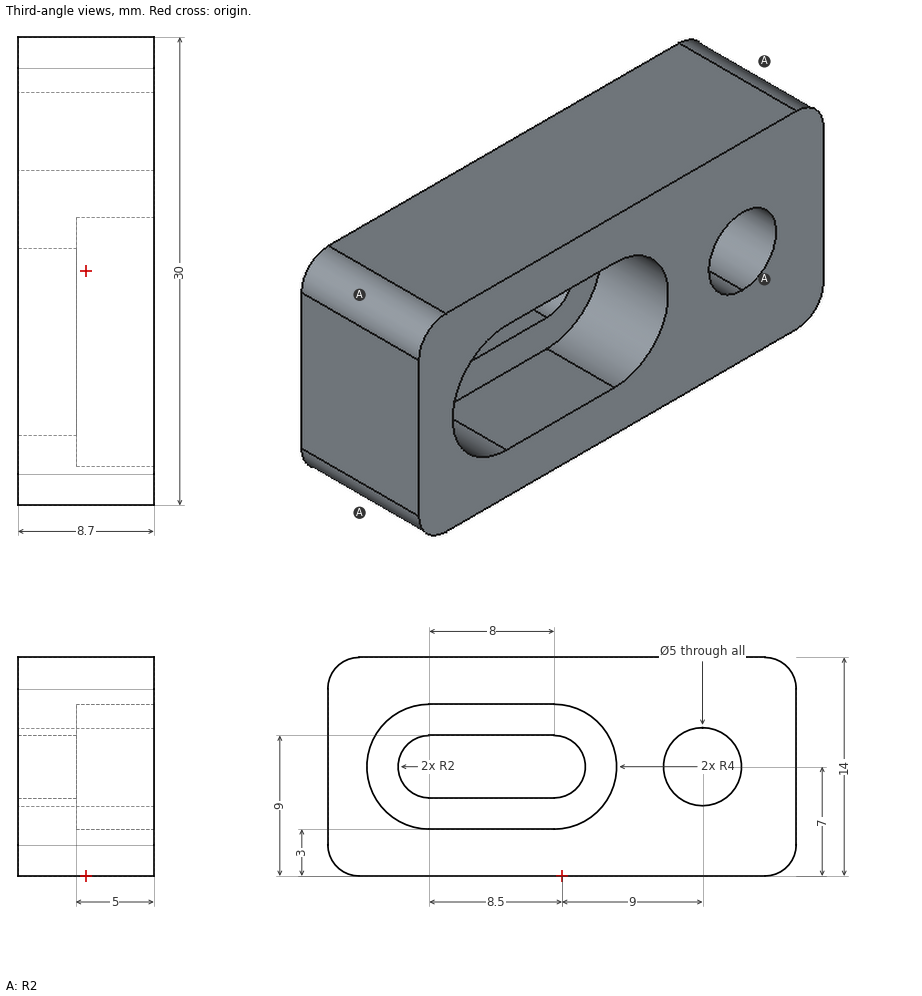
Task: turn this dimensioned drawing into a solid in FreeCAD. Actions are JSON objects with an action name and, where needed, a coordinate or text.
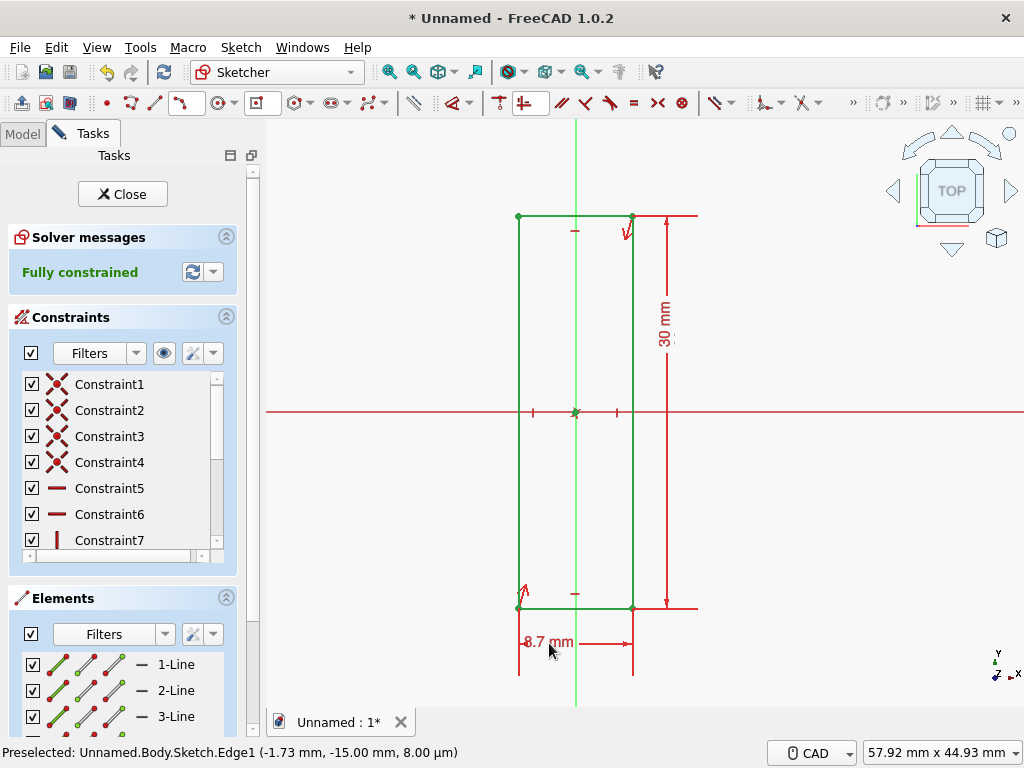
{"action": "left_click", "coordinate": [123, 194]}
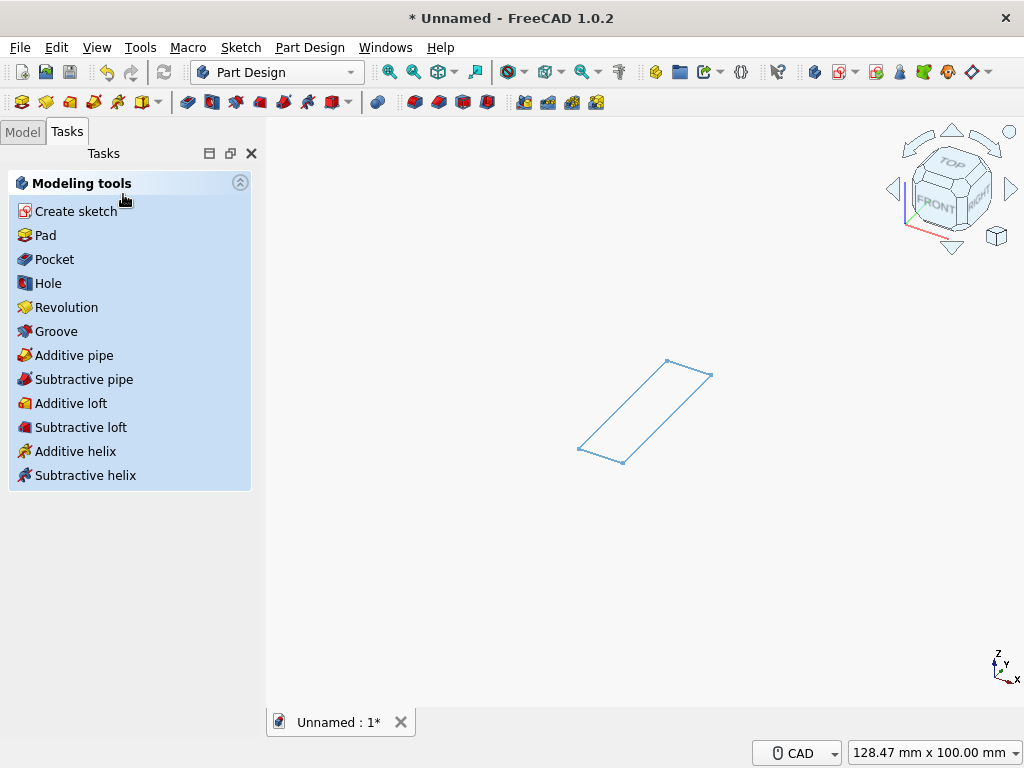
{"action": "left_click", "coordinate": [22, 102]}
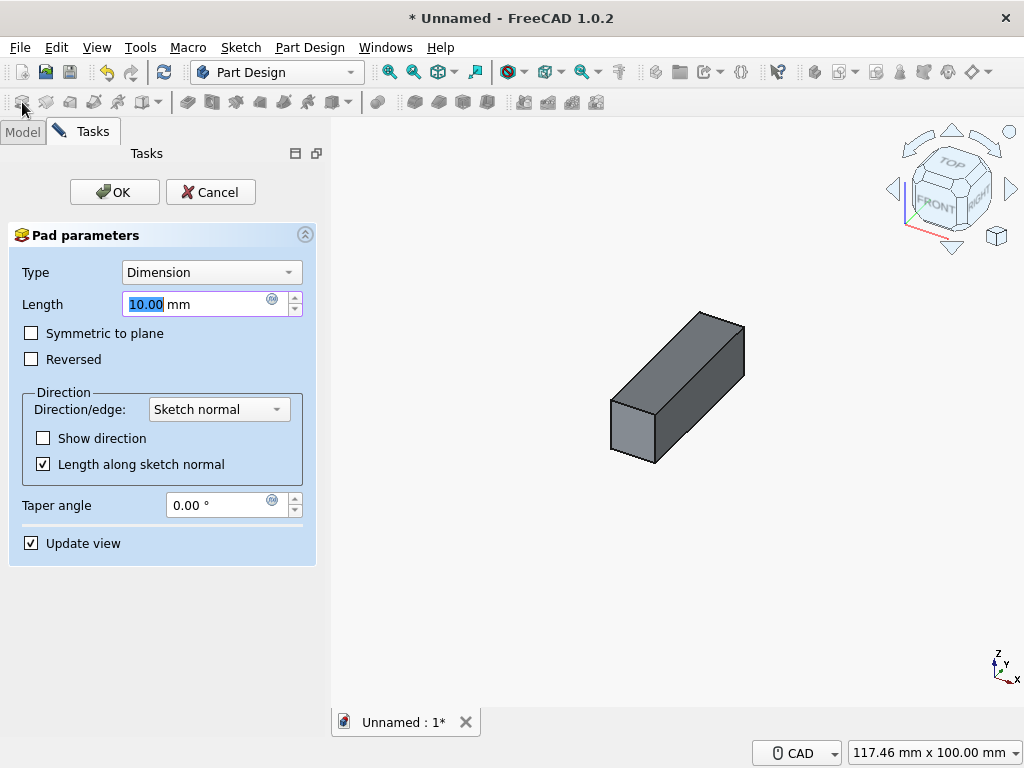
{"action": "type", "text": "14"}
{"action": "key", "text": "Tab"}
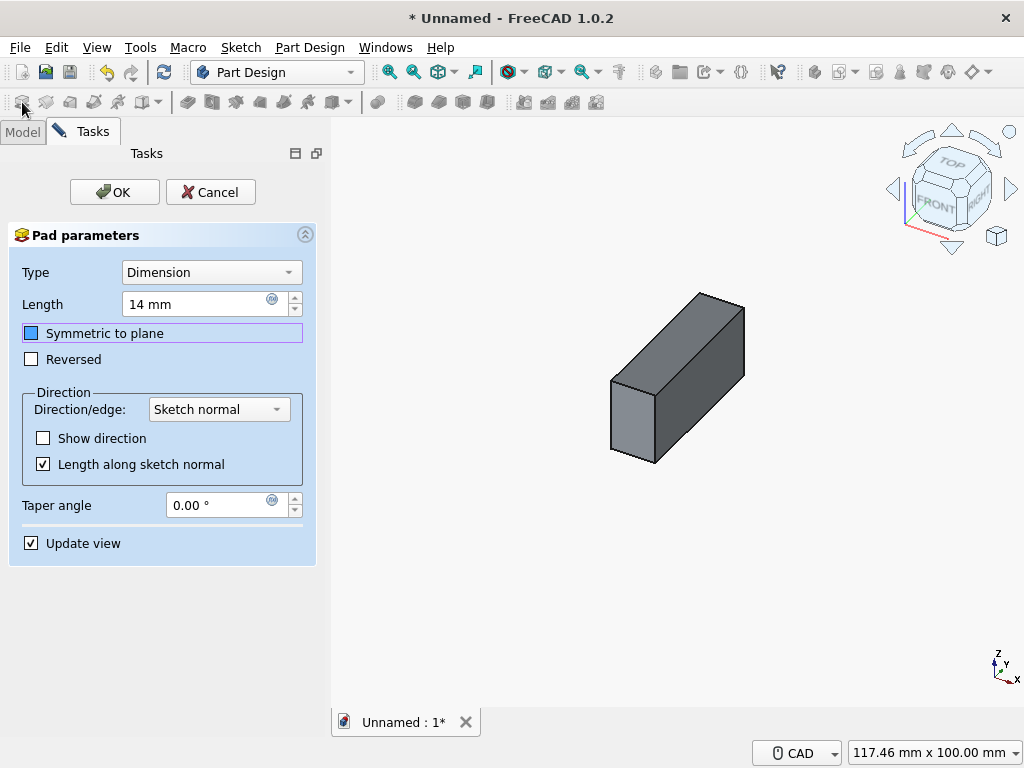
{"action": "left_click", "coordinate": [115, 192]}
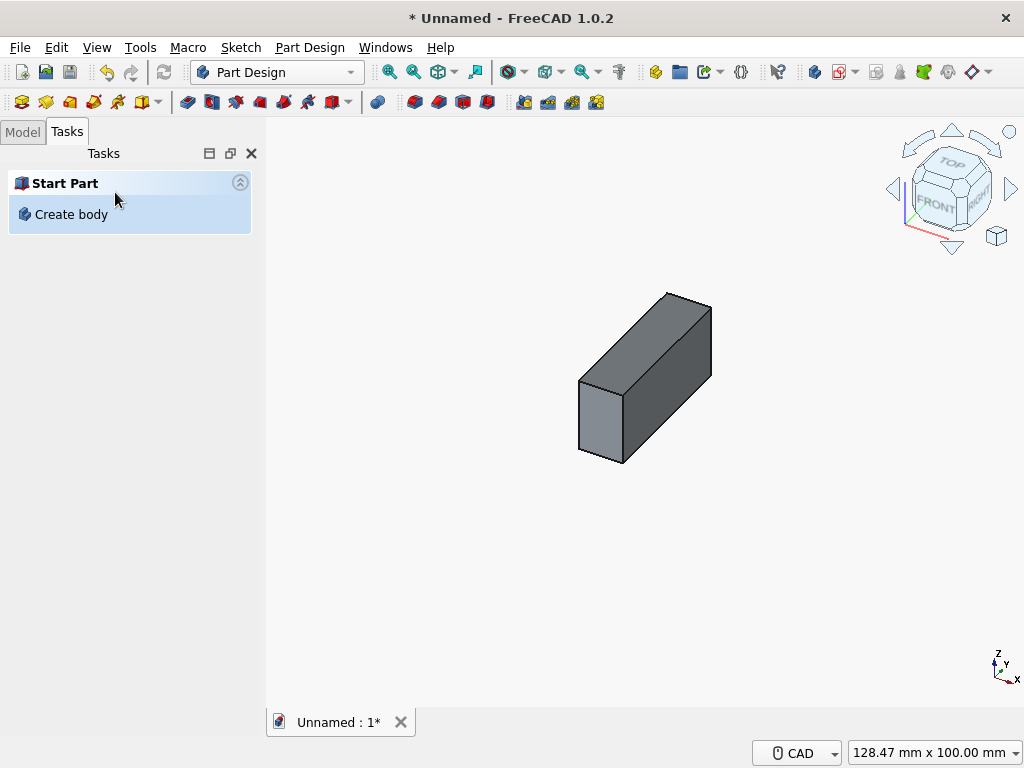
{"action": "left_click", "coordinate": [390, 72]}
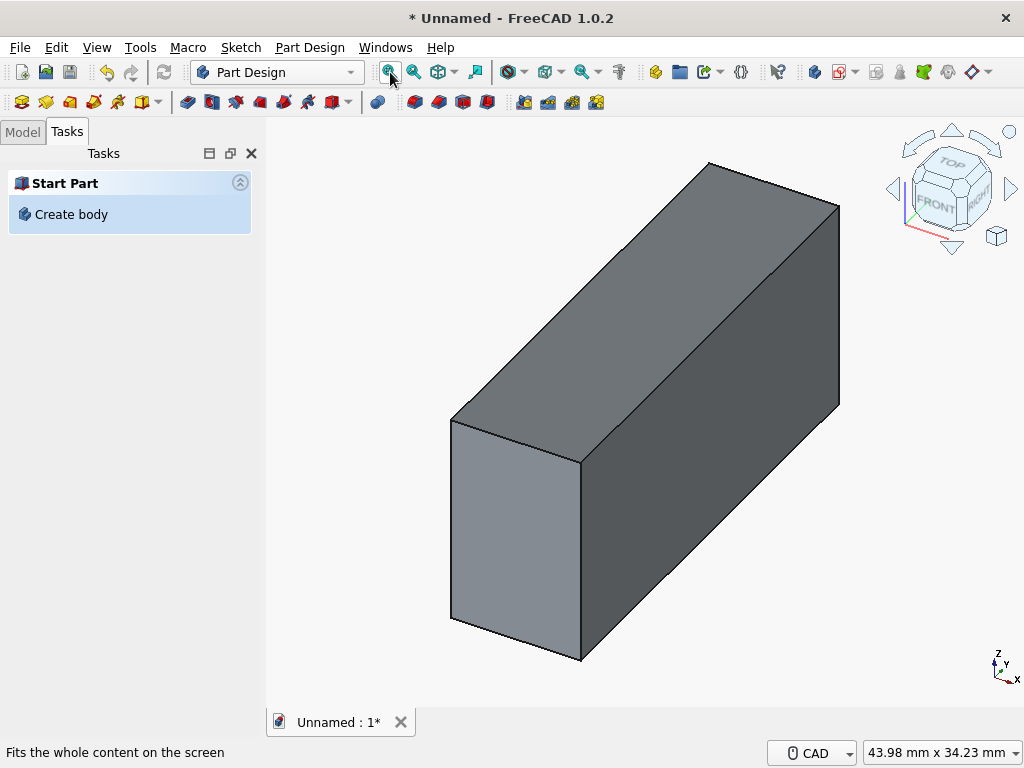
{"action": "left_click", "coordinate": [747, 396]}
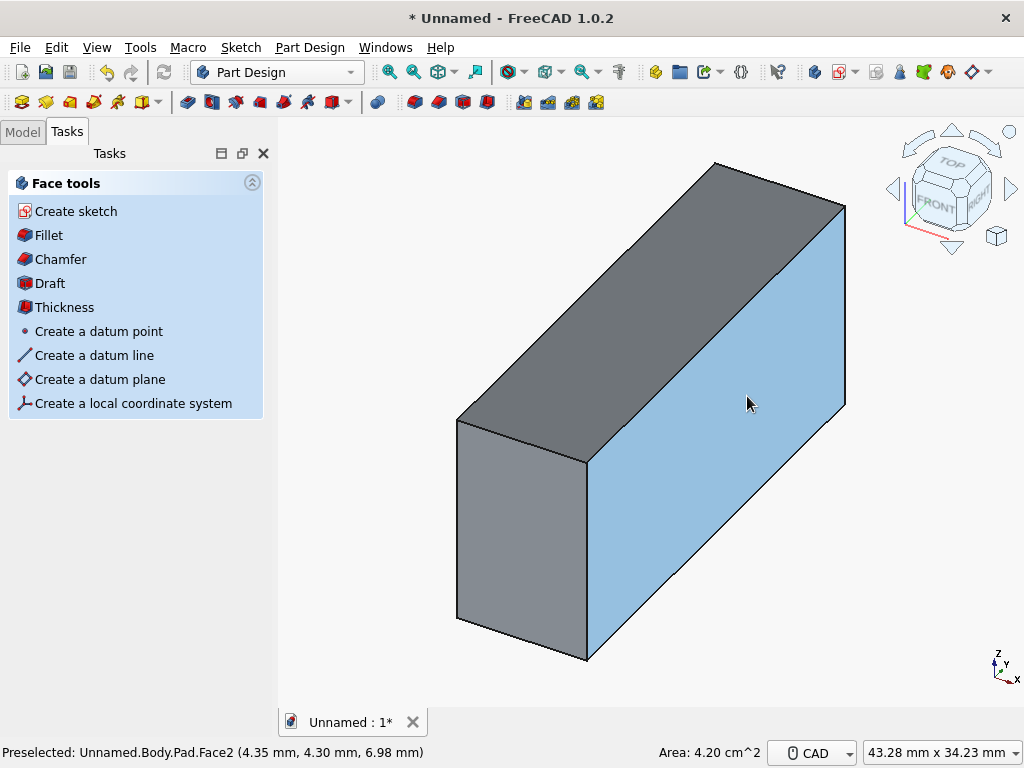
{"action": "left_click", "coordinate": [840, 72]}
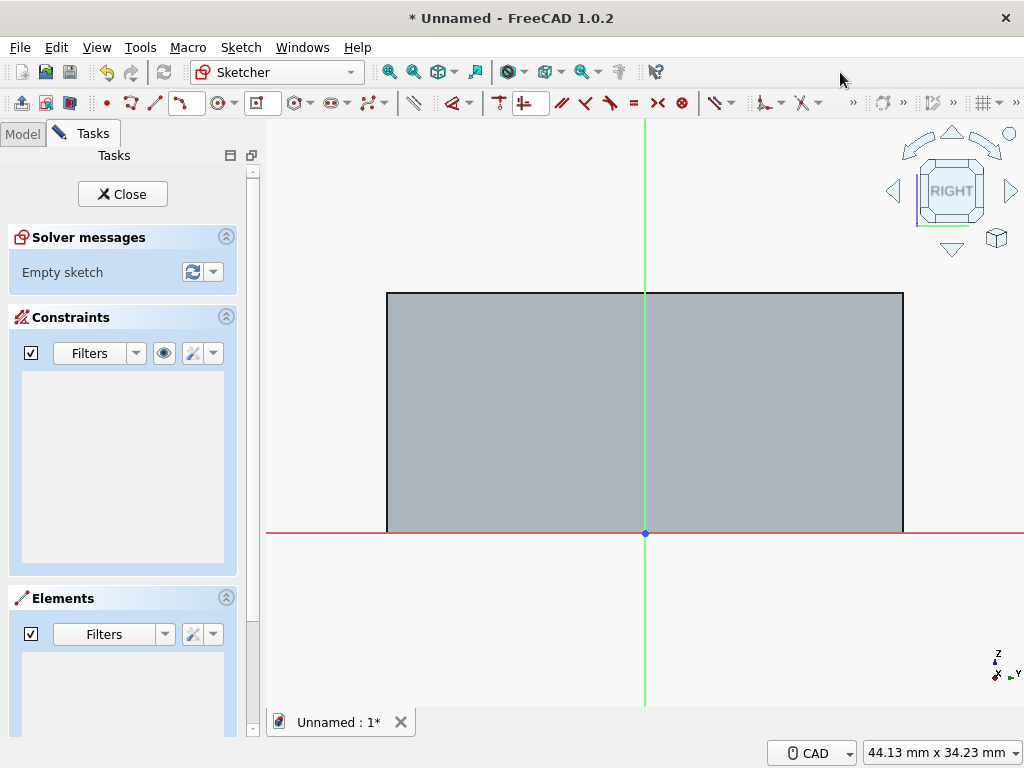
{"action": "scroll", "coordinate": [859, 483], "scroll_direction": "up", "scroll_amount": 4}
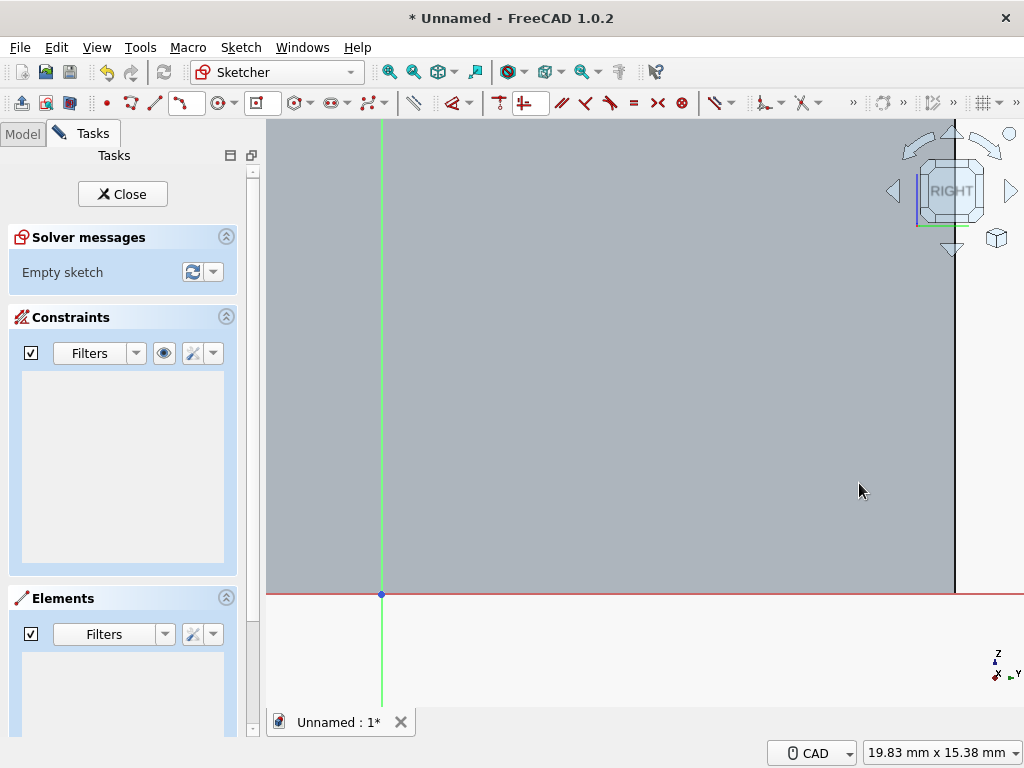
{"action": "left_click", "coordinate": [218, 104]}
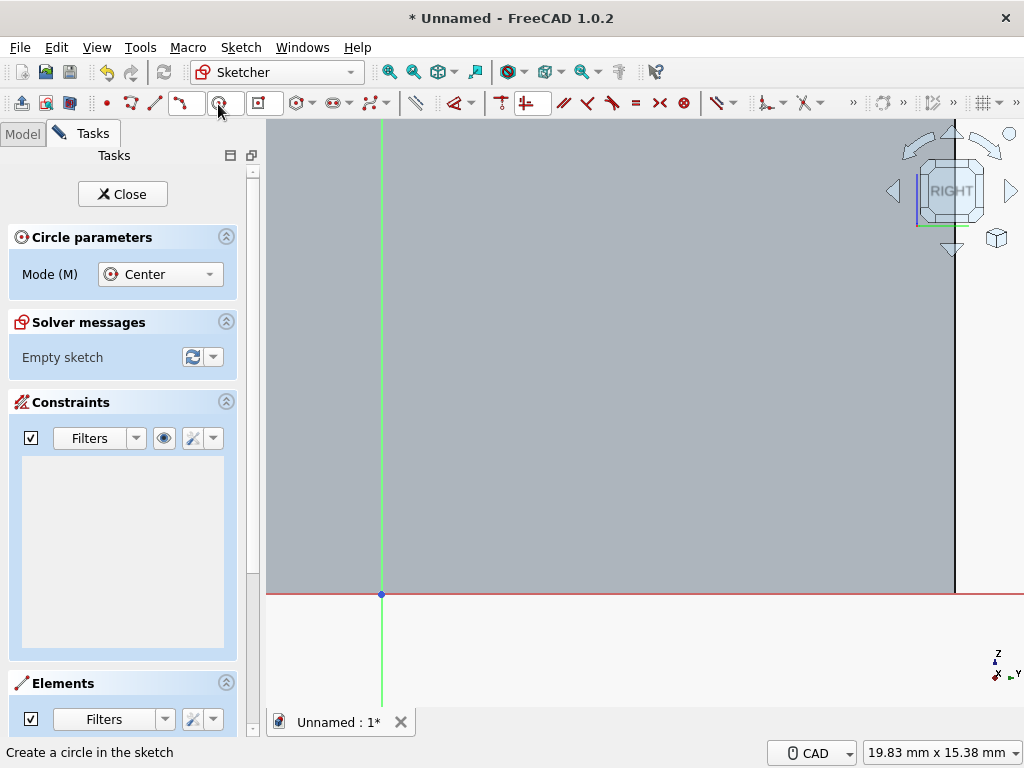
{"action": "left_click", "coordinate": [726, 326]}
{"action": "left_click", "coordinate": [793, 259]}
{"action": "key", "text": "Escape"}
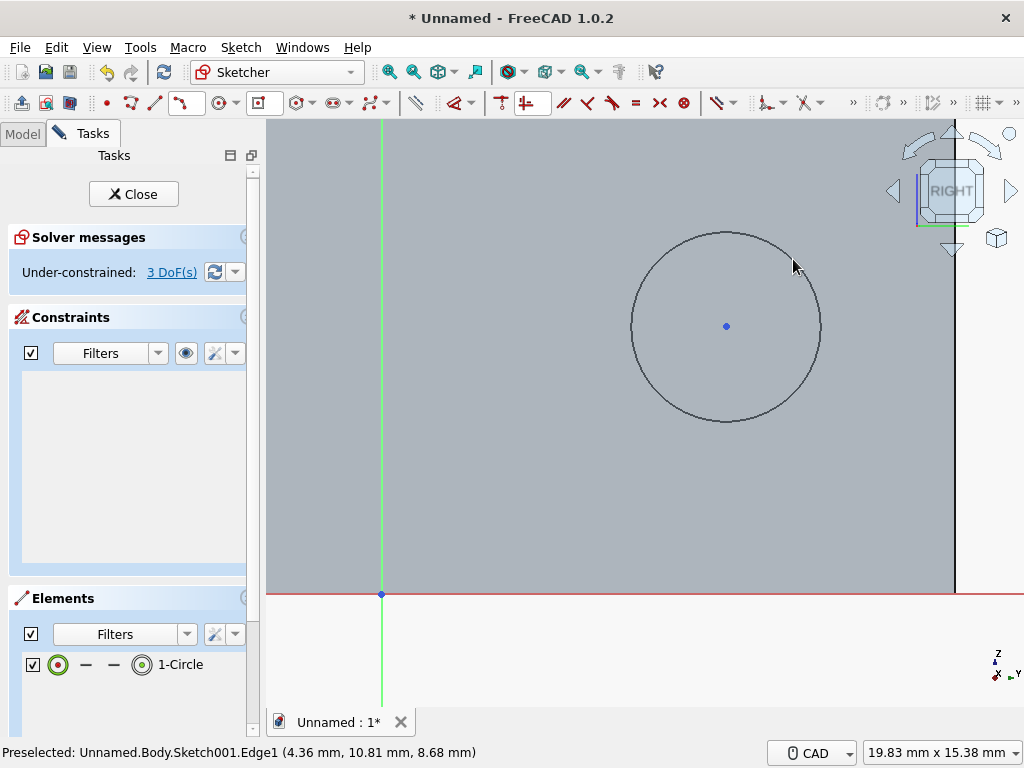
{"action": "left_click", "coordinate": [454, 104]}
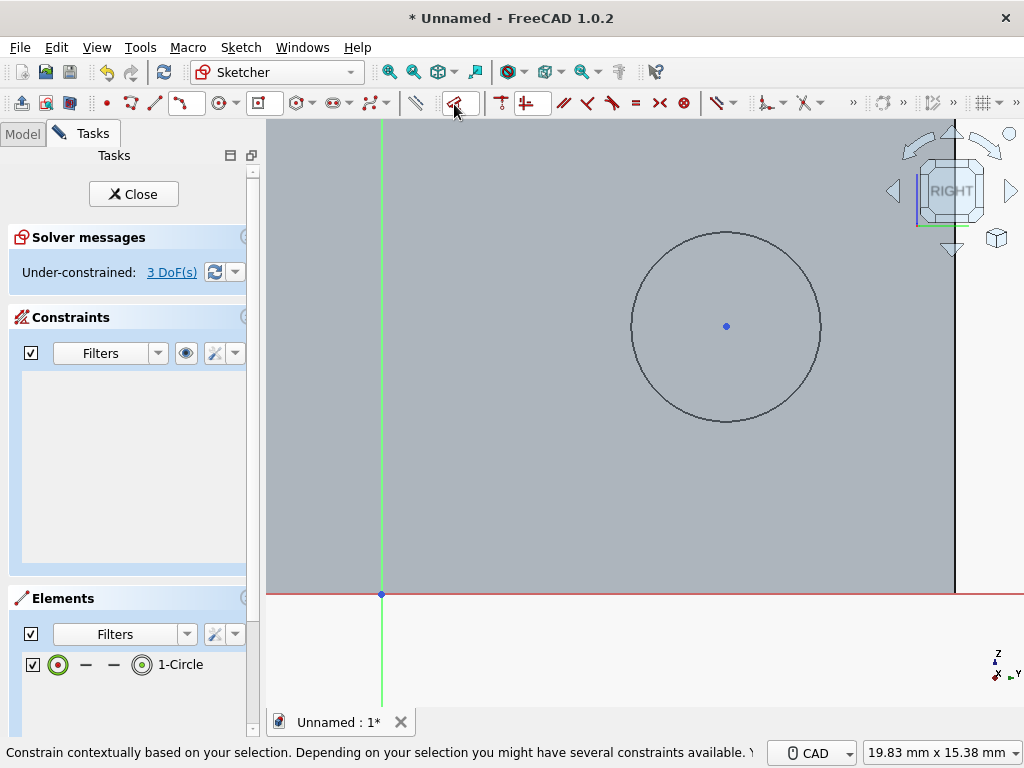
{"action": "left_click", "coordinate": [793, 260]}
{"action": "left_click", "coordinate": [816, 237]}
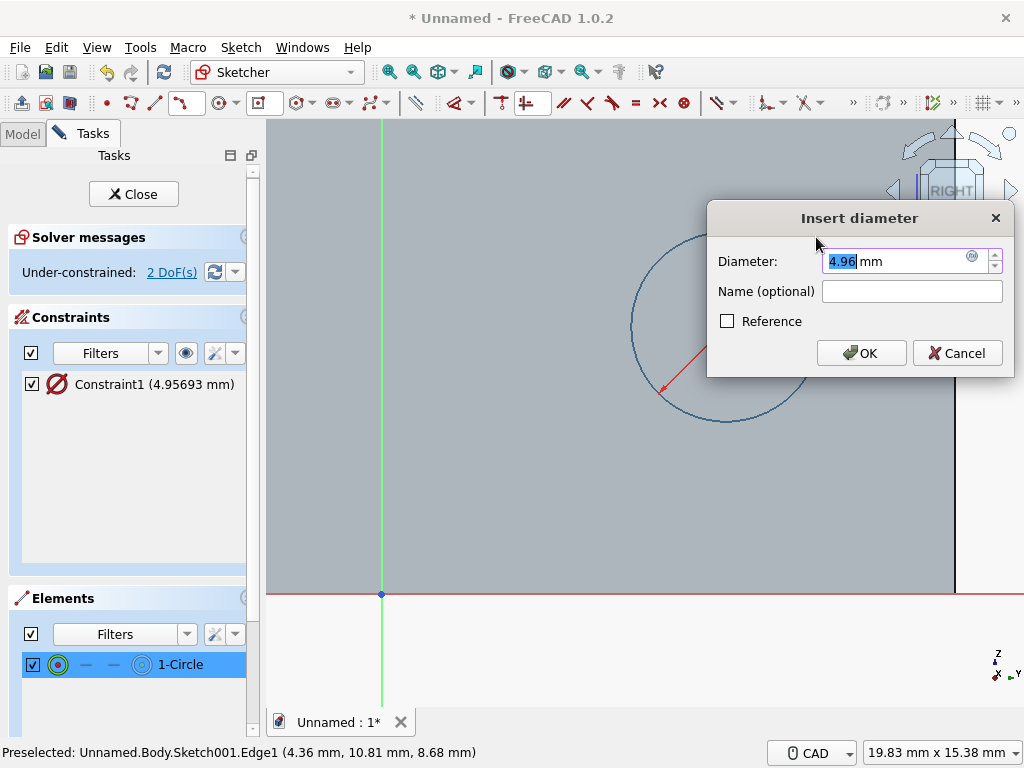
{"action": "type", "text": "5"}
{"action": "key", "text": "Return"}